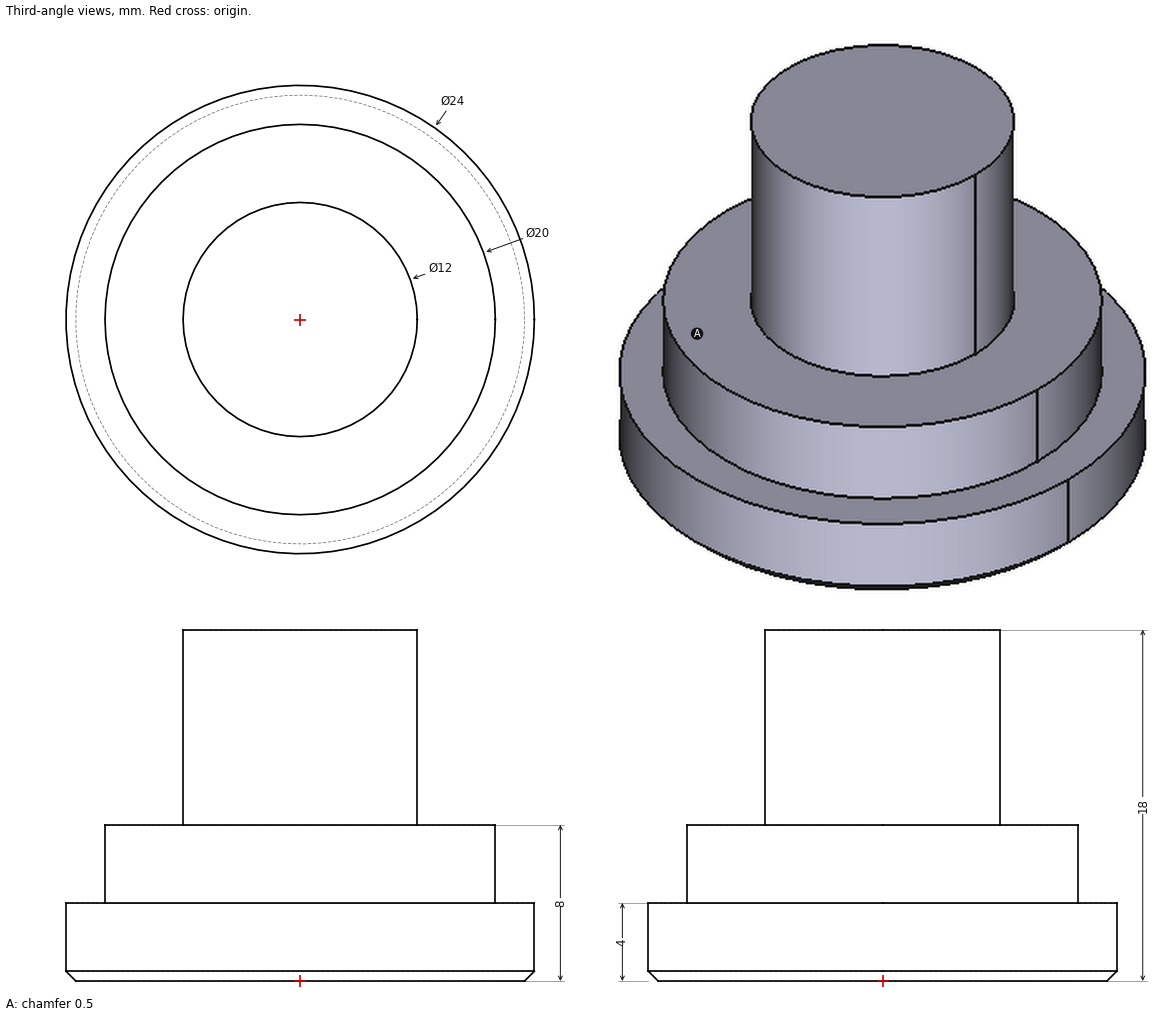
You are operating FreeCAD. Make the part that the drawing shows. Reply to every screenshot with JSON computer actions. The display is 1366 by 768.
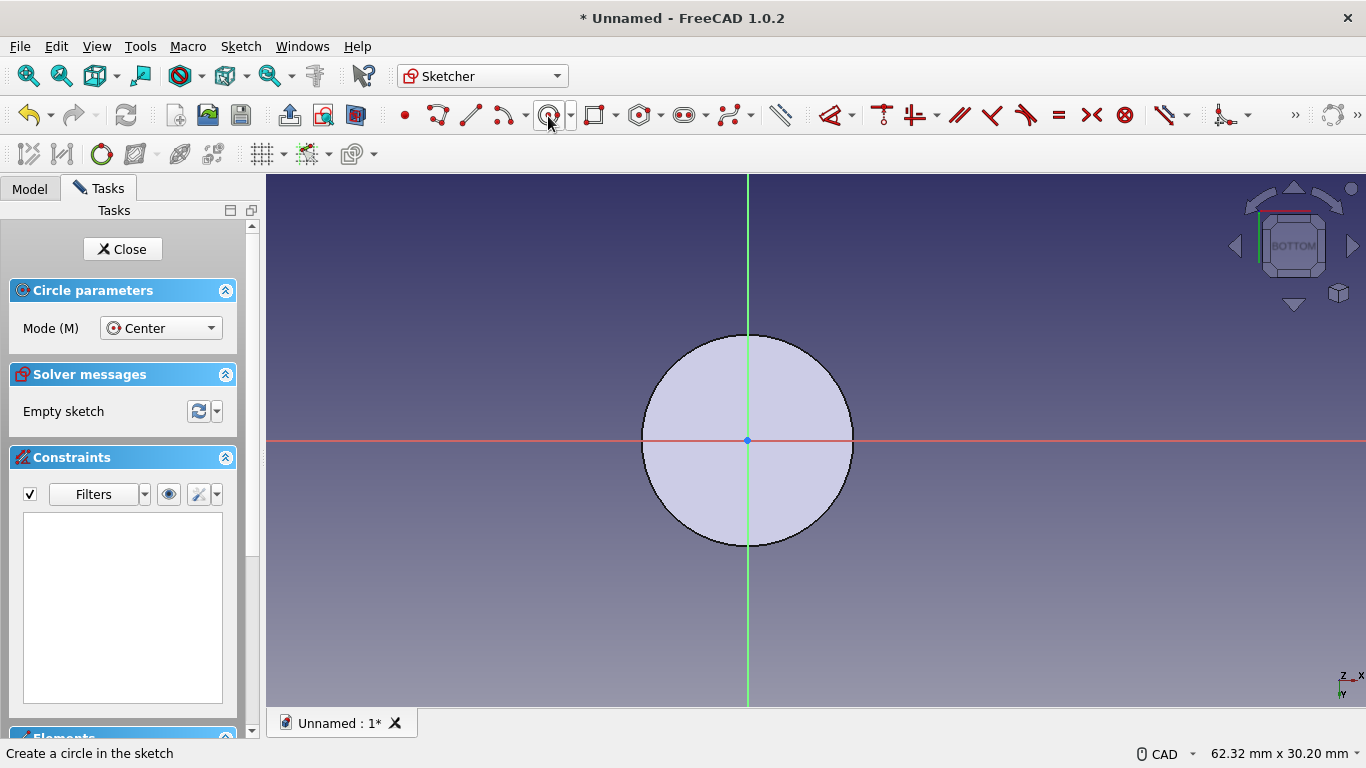
{"action": "left_click", "coordinate": [748, 440]}
{"action": "mouse_move", "coordinate": [872, 316]}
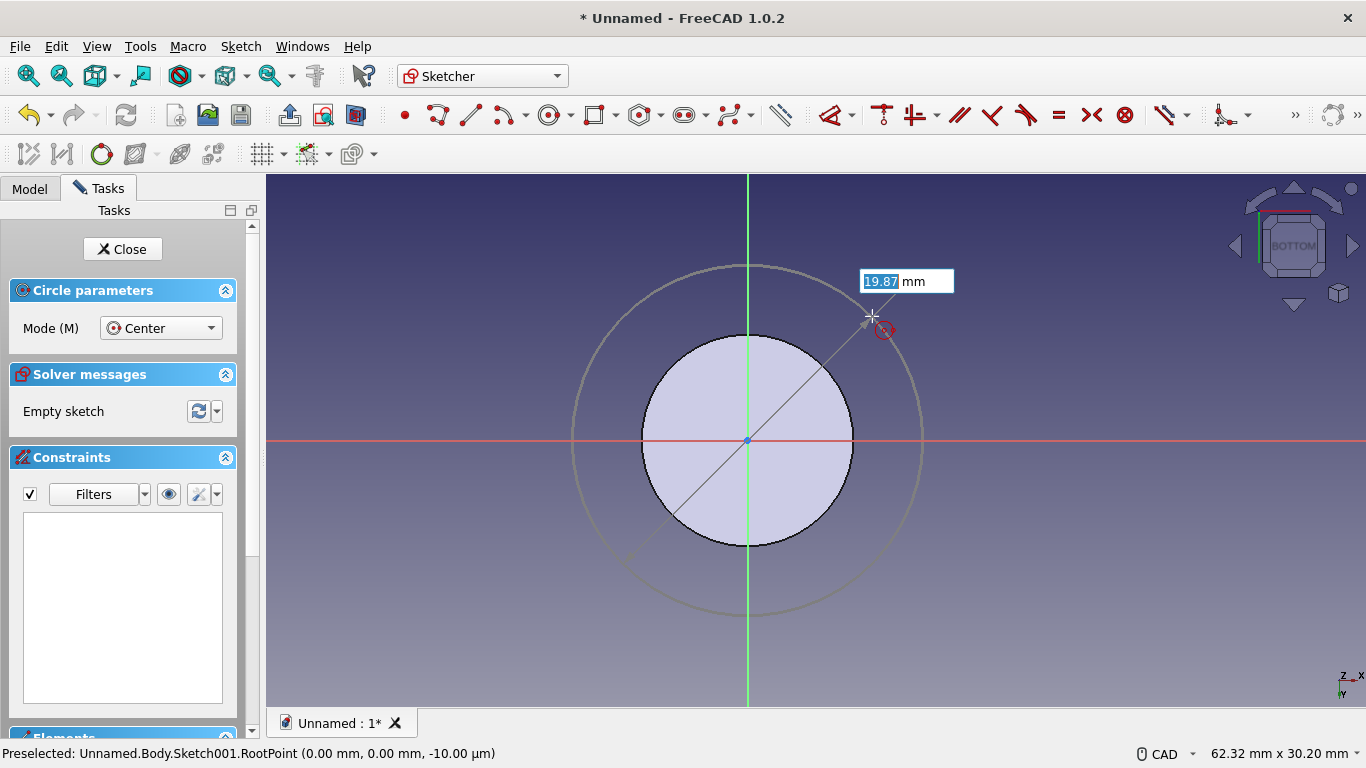
{"action": "type", "text": "20"}
{"action": "key", "text": "Return"}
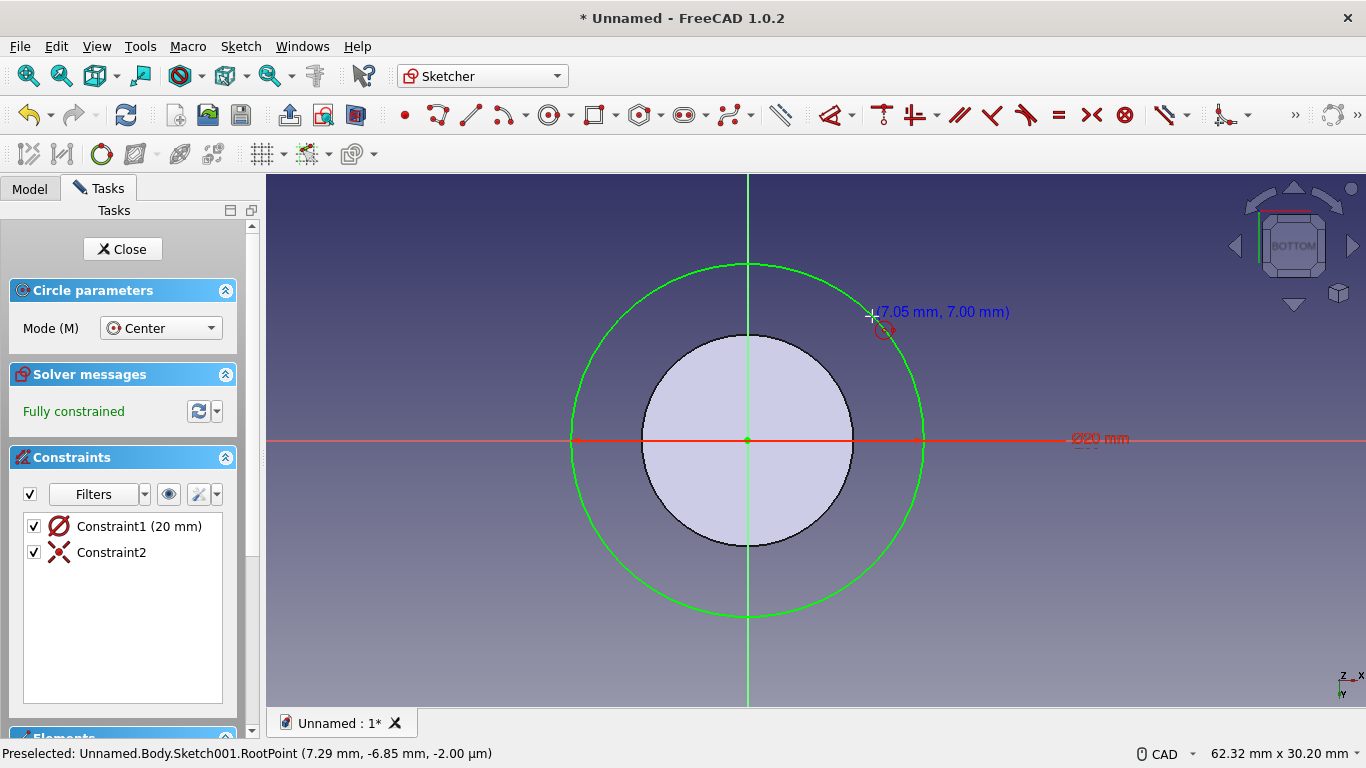
{"action": "left_click", "coordinate": [748, 440]}
{"action": "mouse_move", "coordinate": [822, 366]}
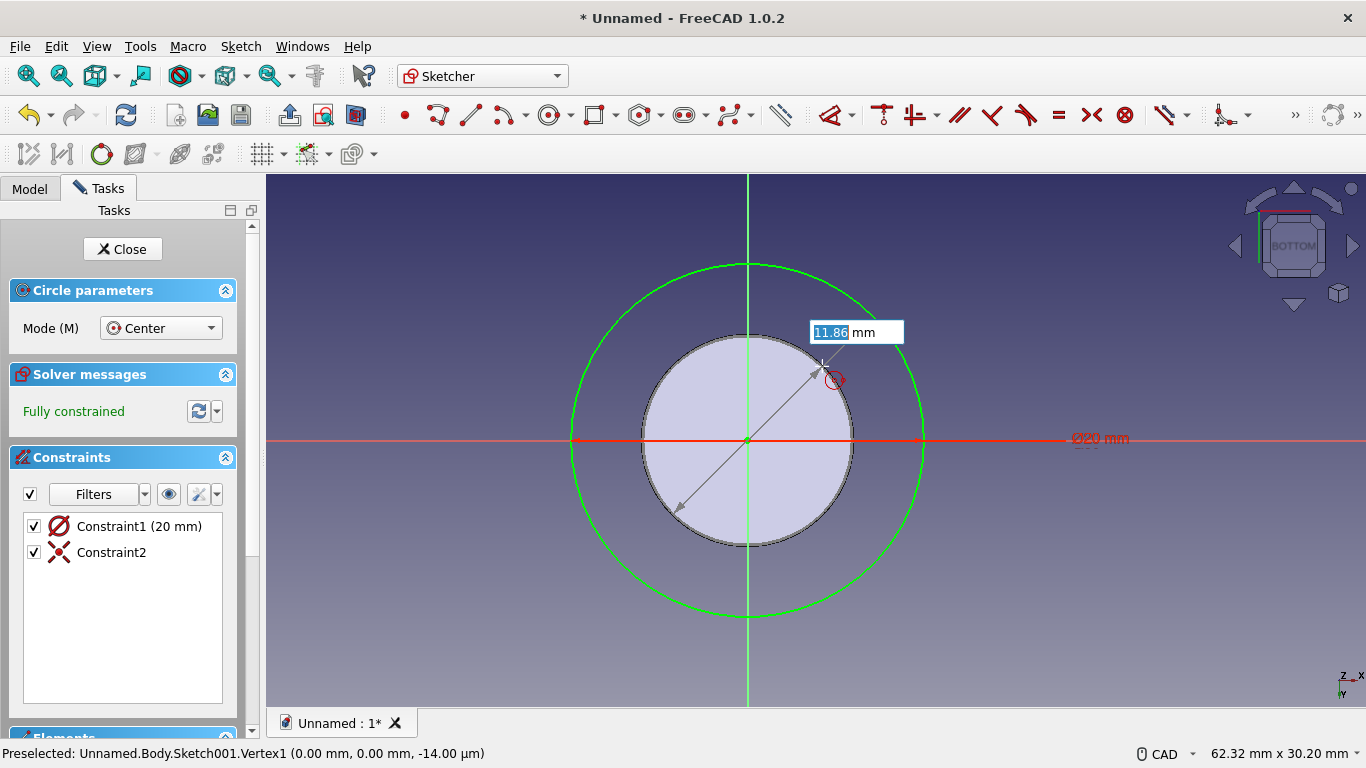
{"action": "type", "text": "12"}
{"action": "key", "text": "Return"}
{"action": "key", "text": "Escape"}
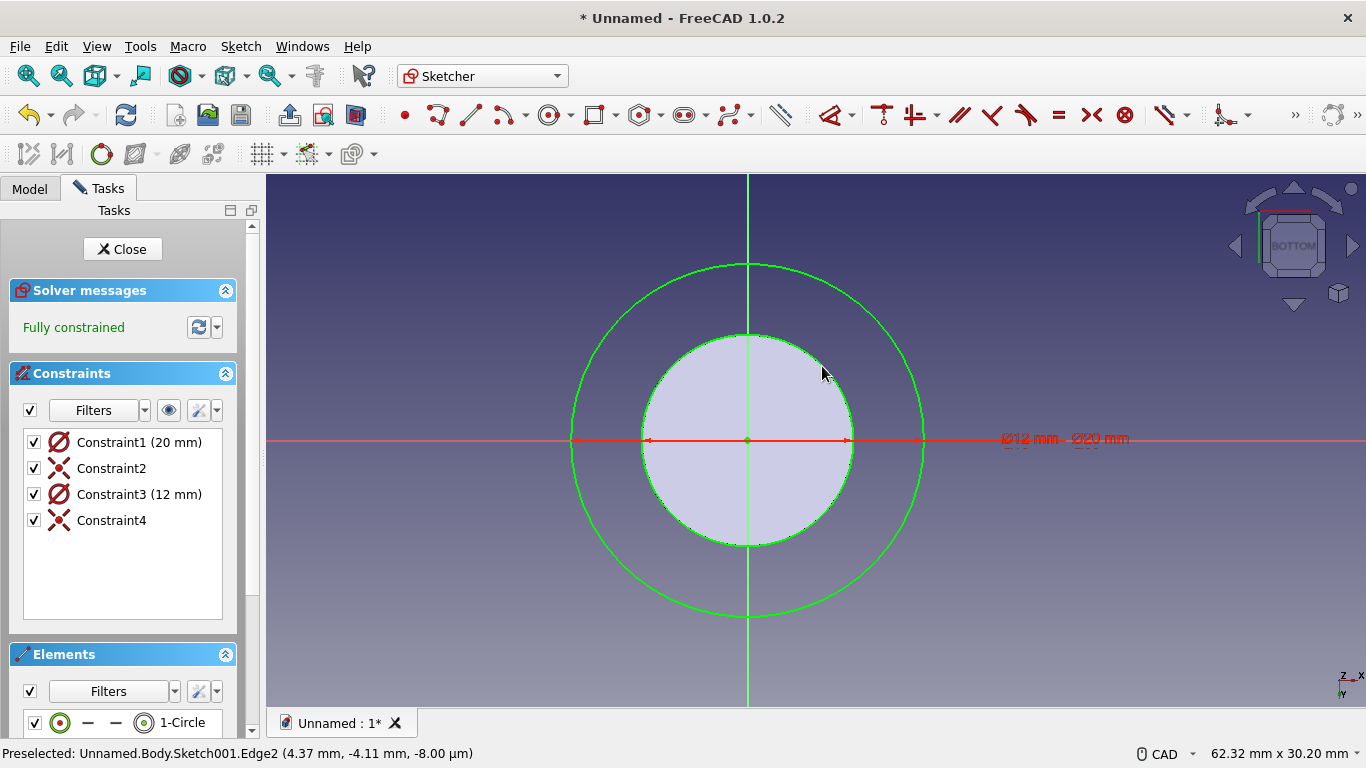
{"action": "left_click", "coordinate": [123, 249]}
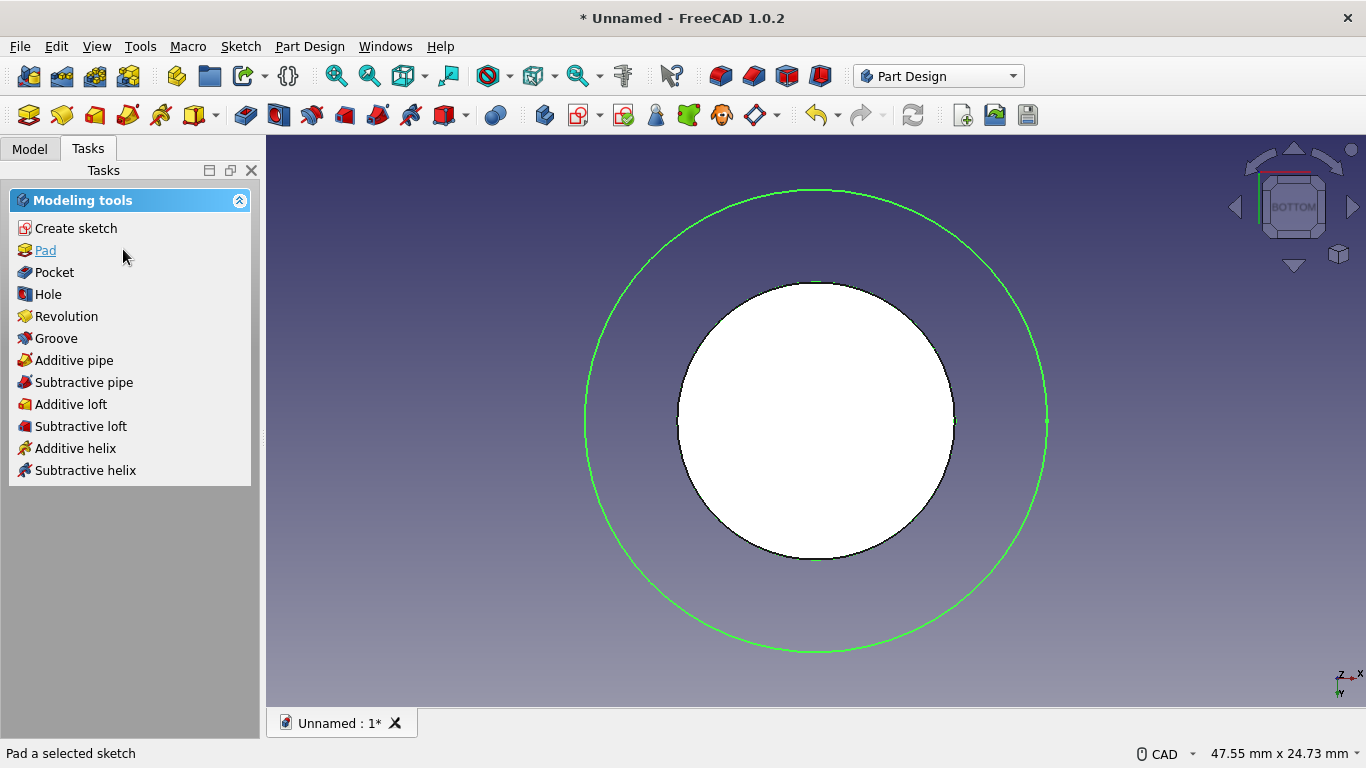
{"action": "left_click", "coordinate": [29, 116]}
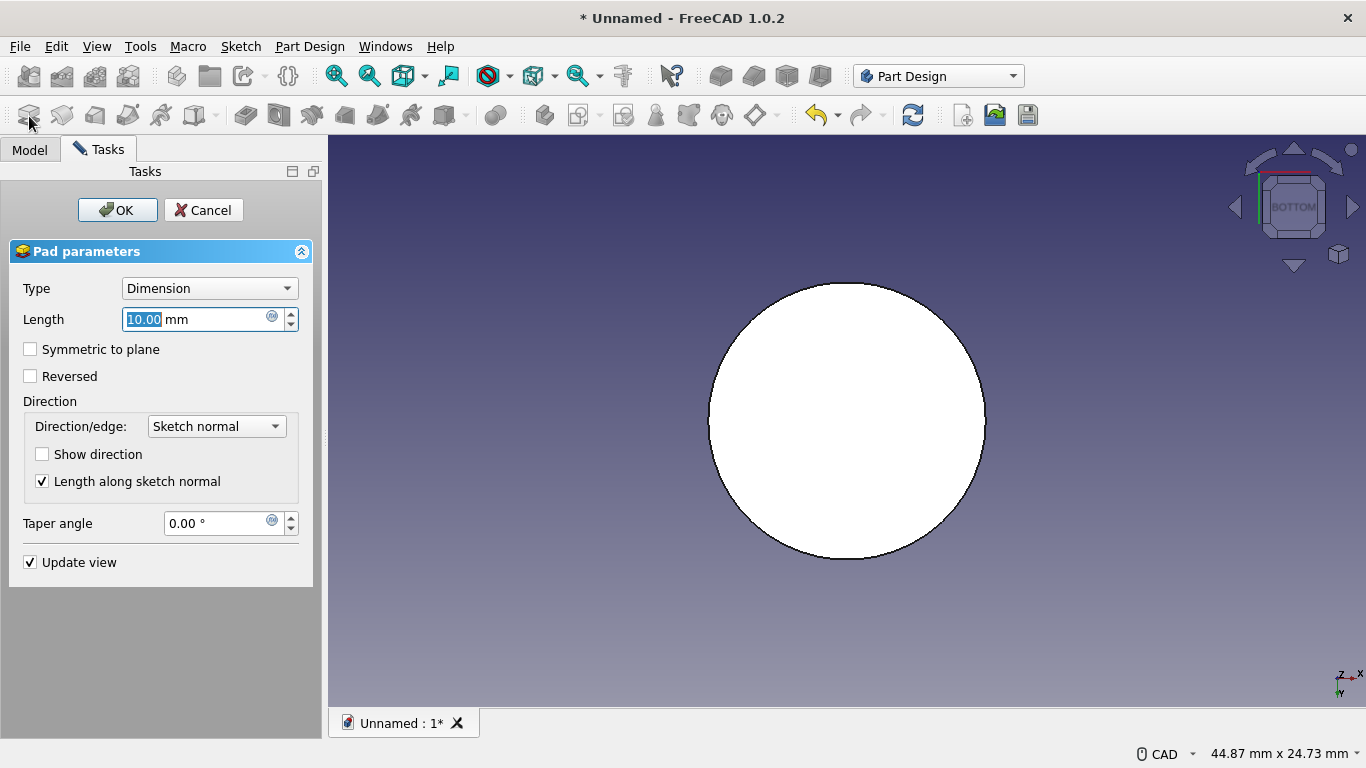
{"action": "type", "text": "8"}
{"action": "key", "text": "Tab"}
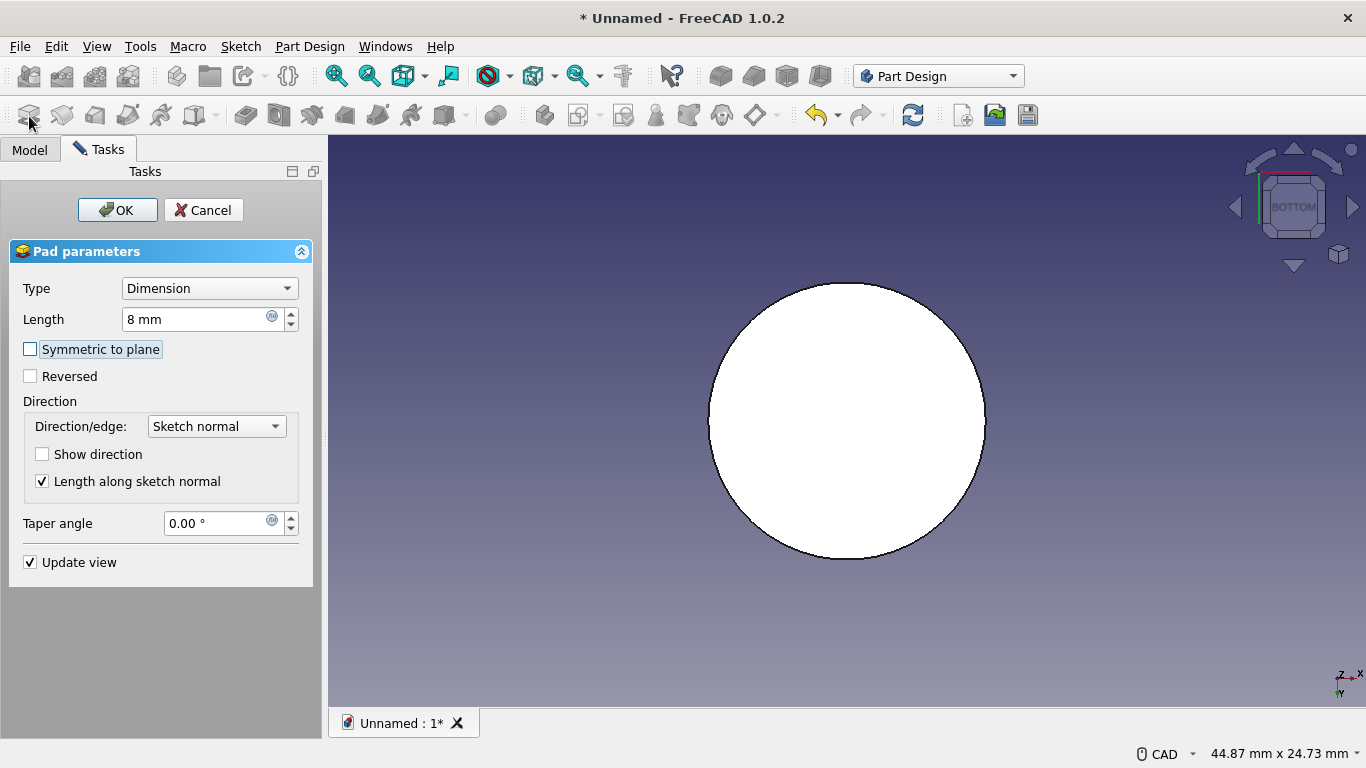
{"action": "left_click", "coordinate": [31, 376]}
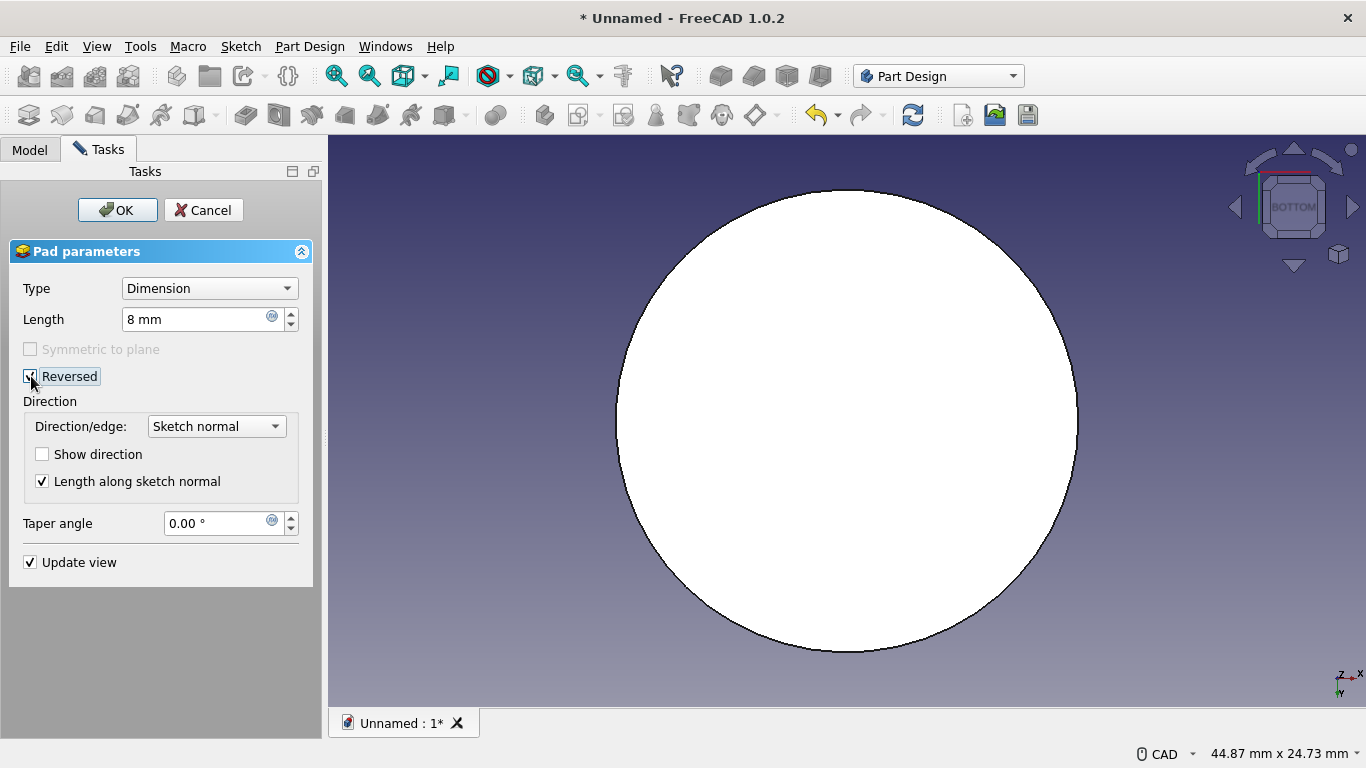
{"action": "left_click", "coordinate": [118, 210]}